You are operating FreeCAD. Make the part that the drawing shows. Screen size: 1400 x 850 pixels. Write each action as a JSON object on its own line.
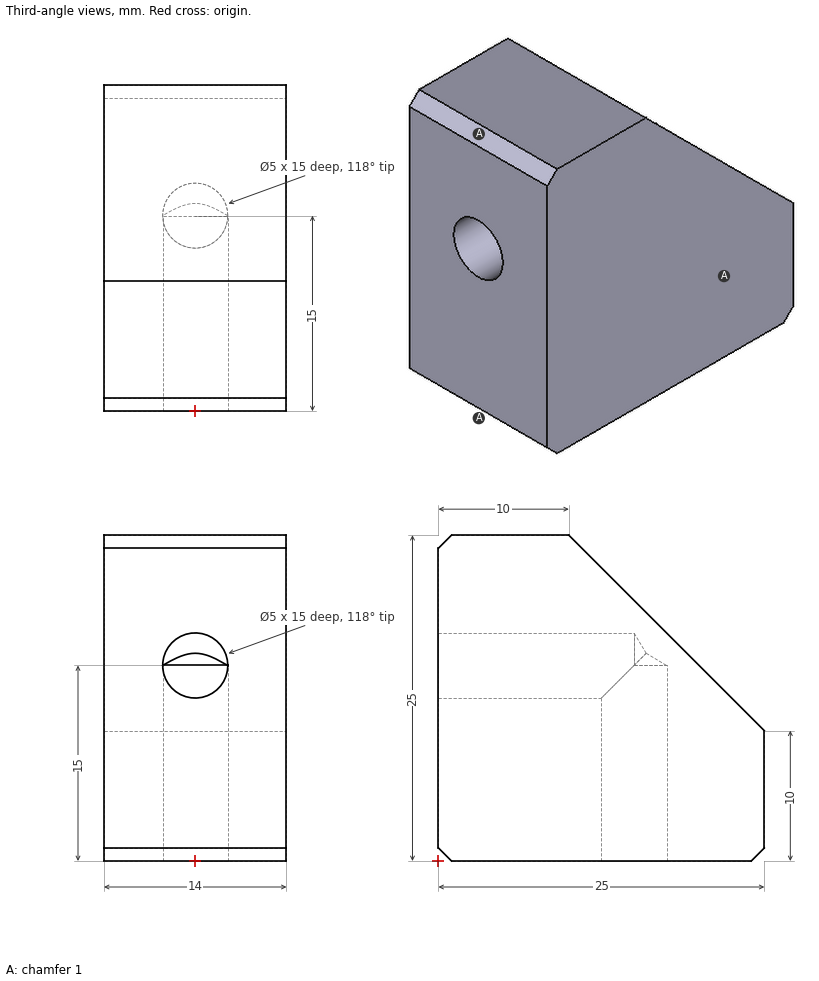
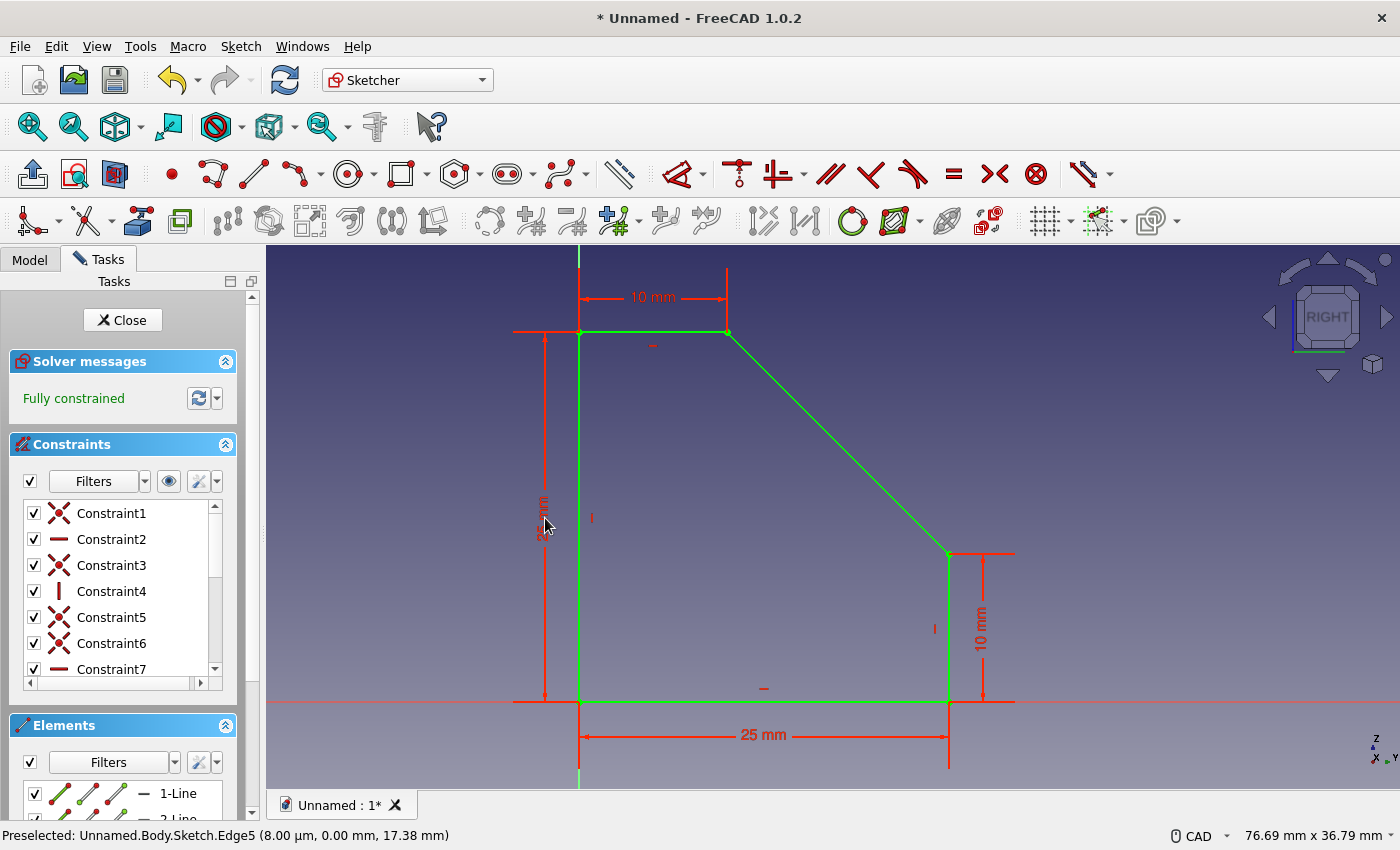
{"action": "left_click", "coordinate": [123, 320]}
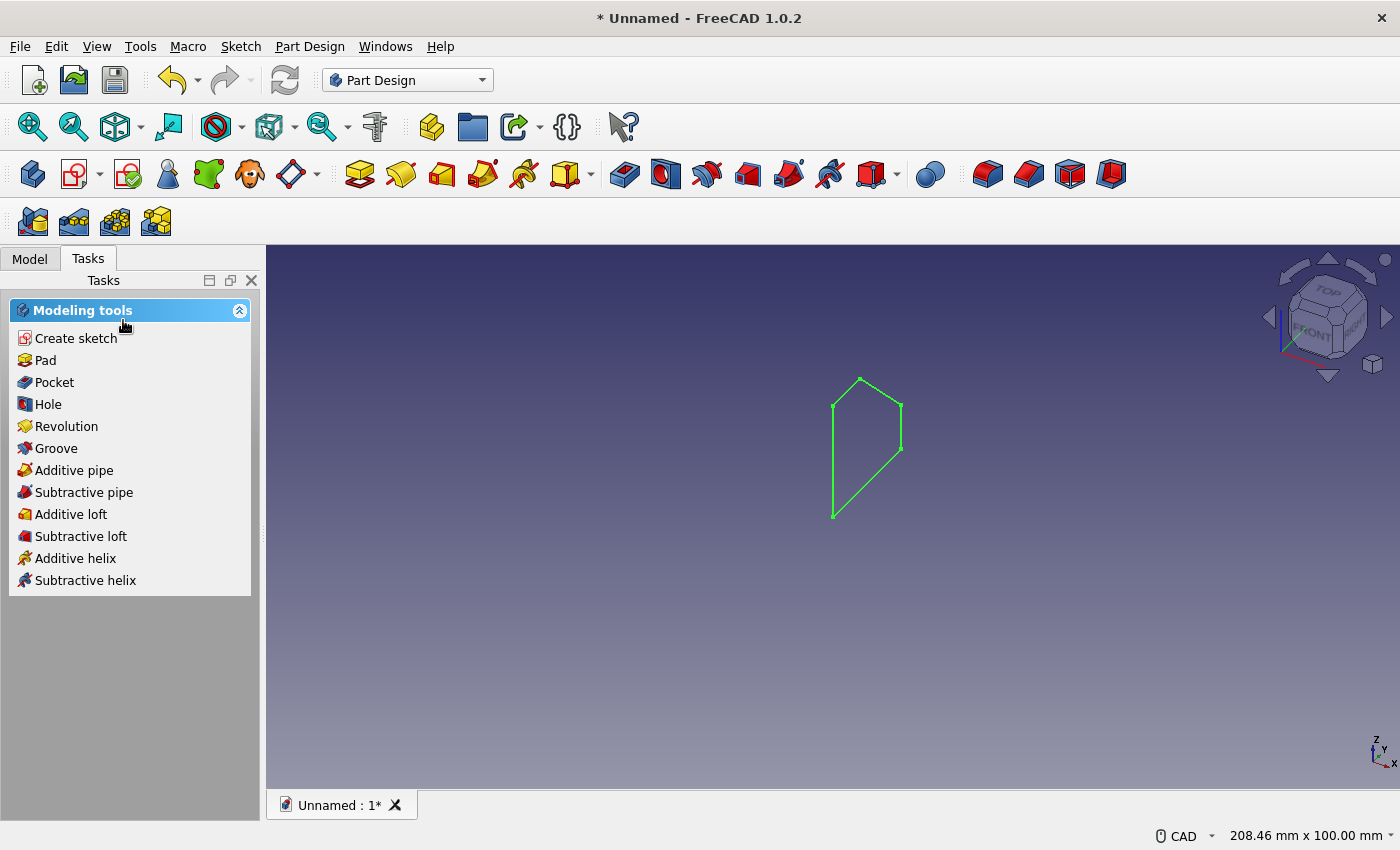
{"action": "left_click", "coordinate": [360, 174]}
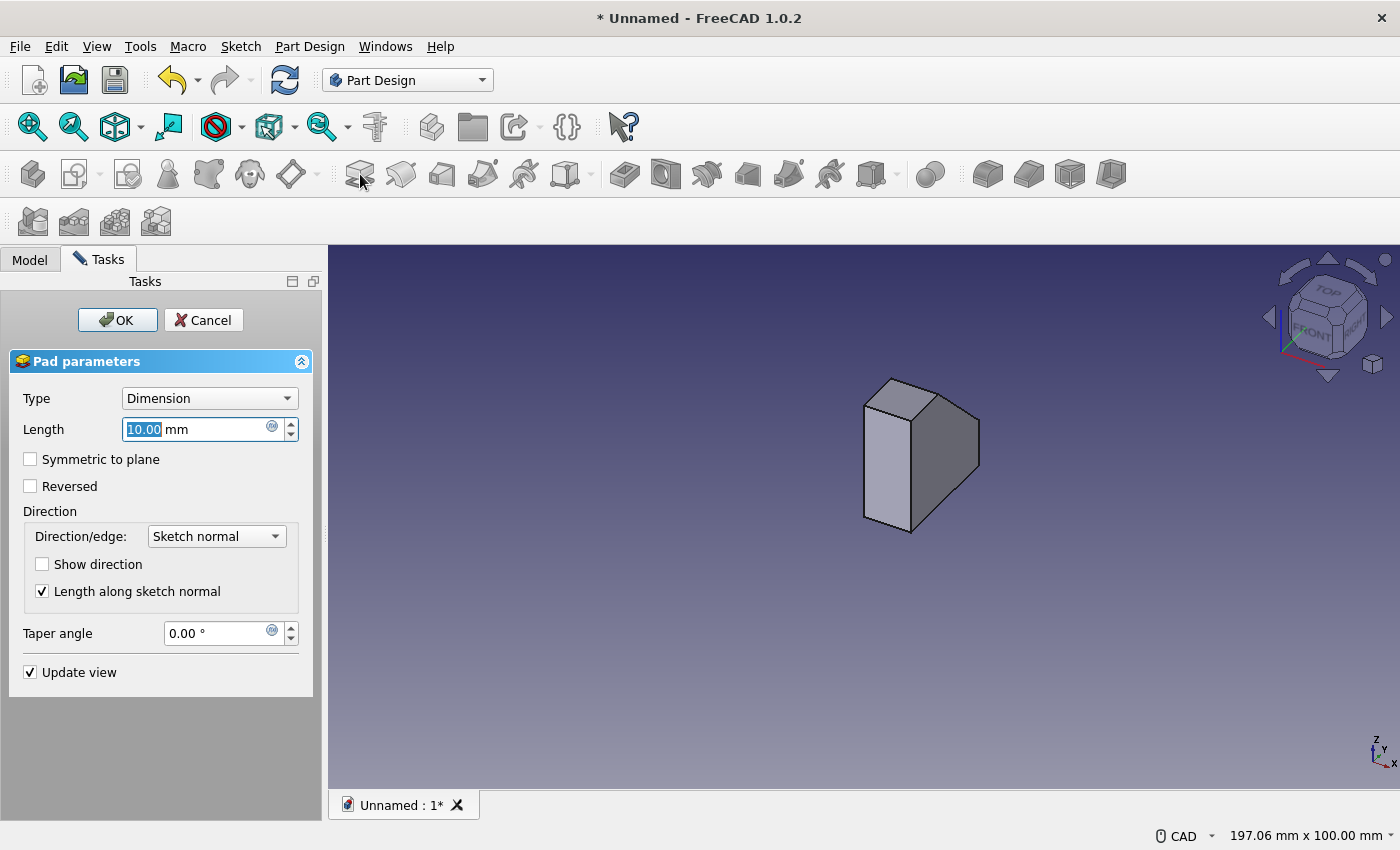
{"action": "type", "text": "14"}
{"action": "key", "text": "Tab"}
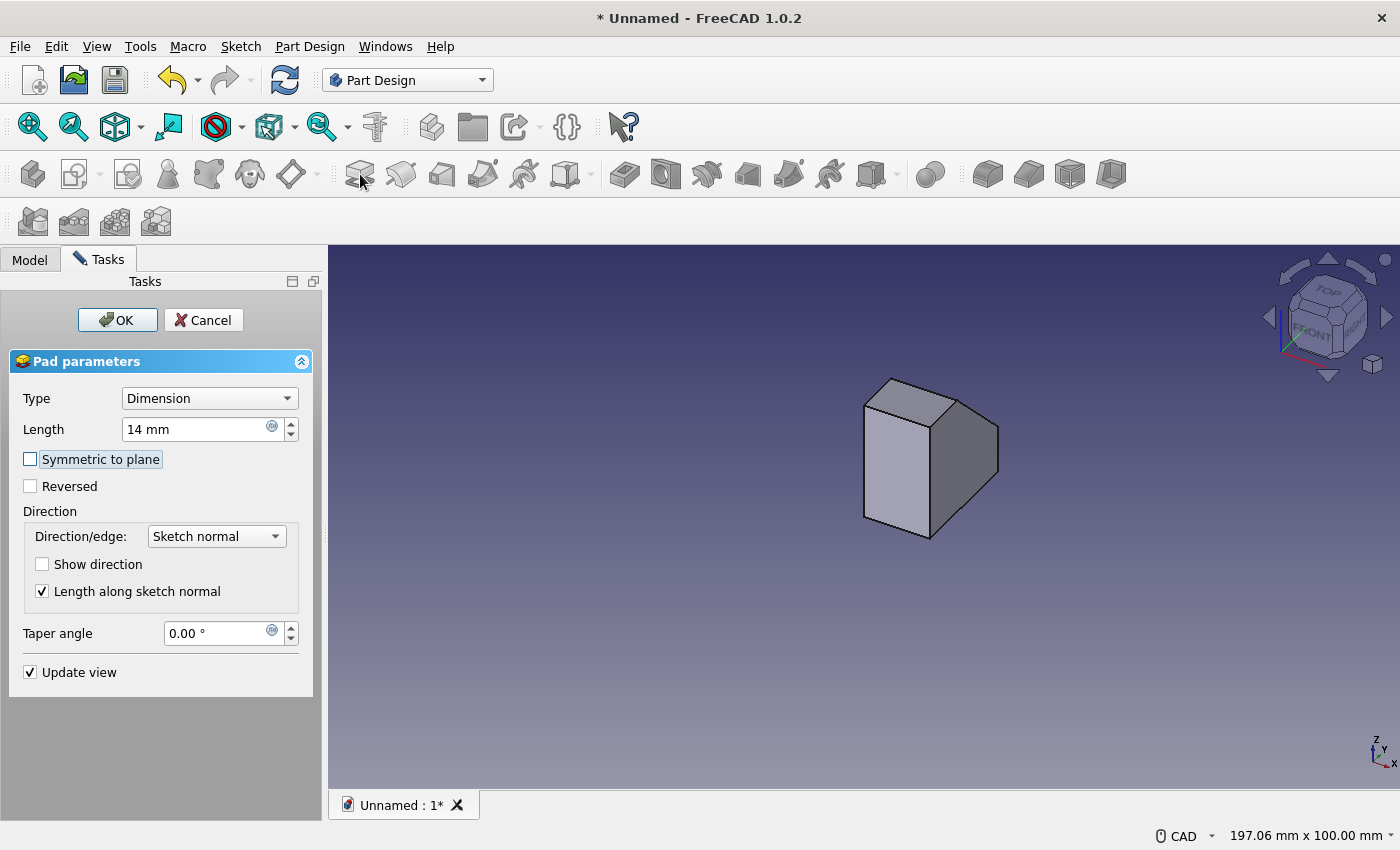
{"action": "left_click", "coordinate": [31, 459]}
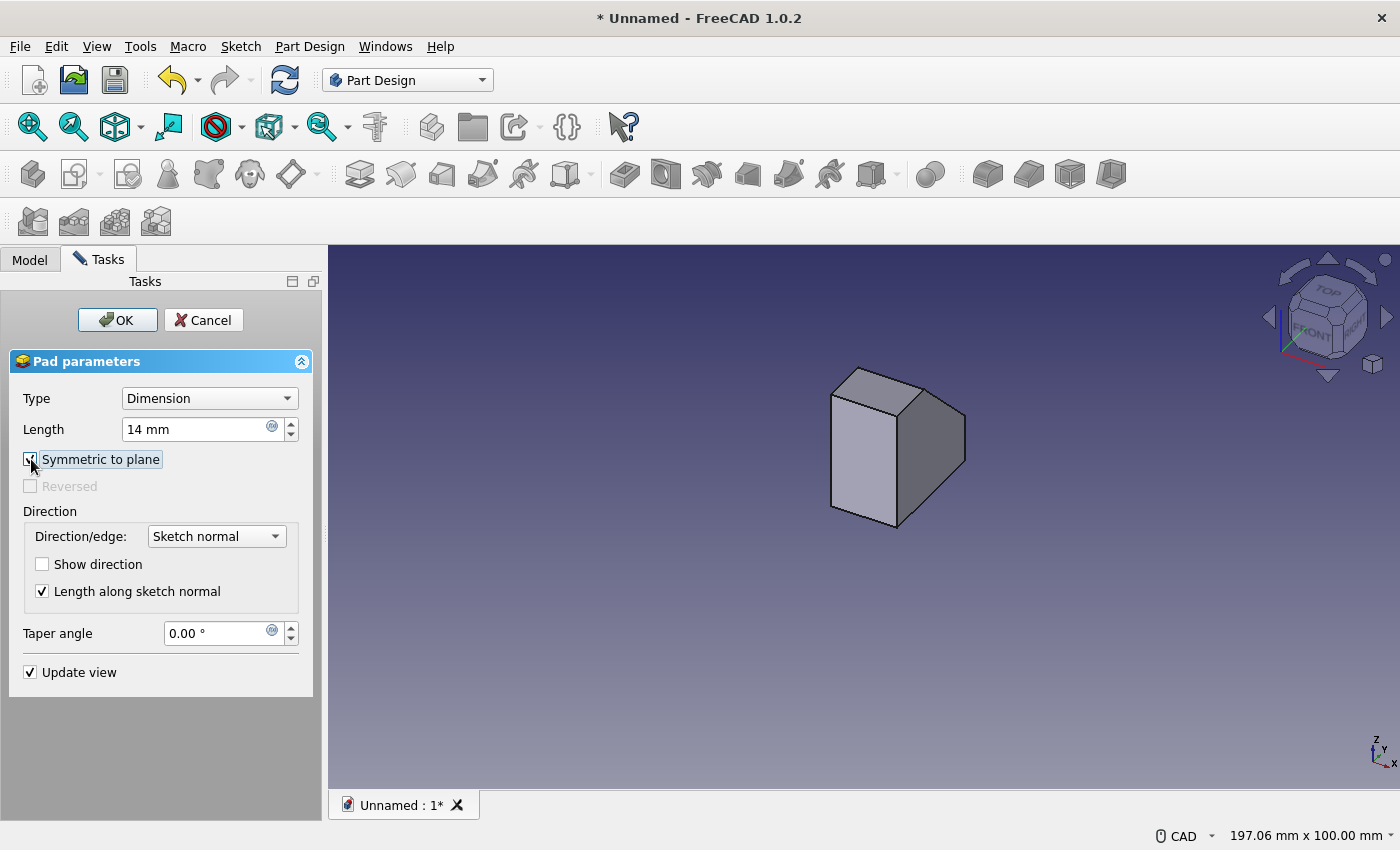
{"action": "left_click", "coordinate": [118, 320]}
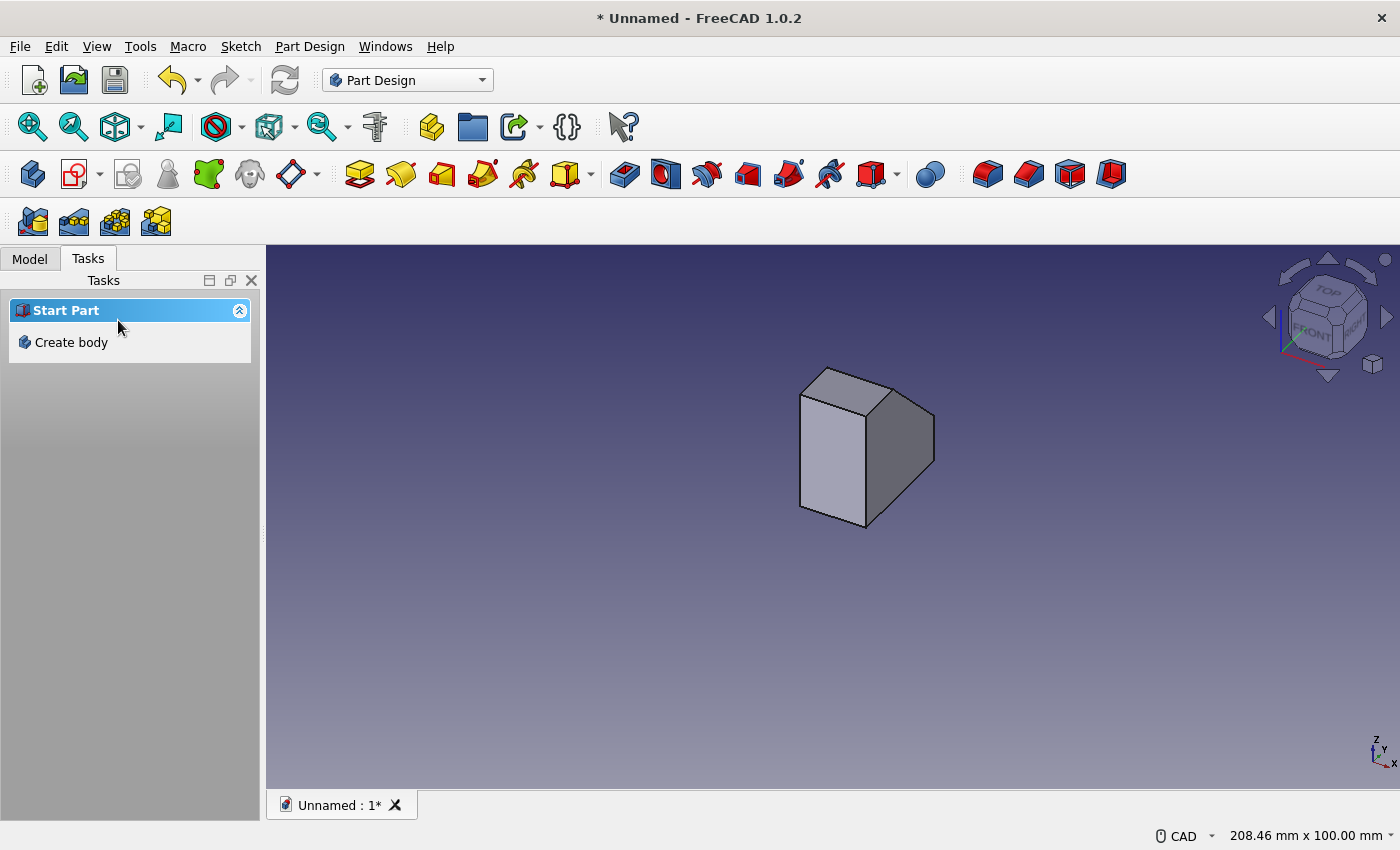
{"action": "left_click", "coordinate": [33, 128]}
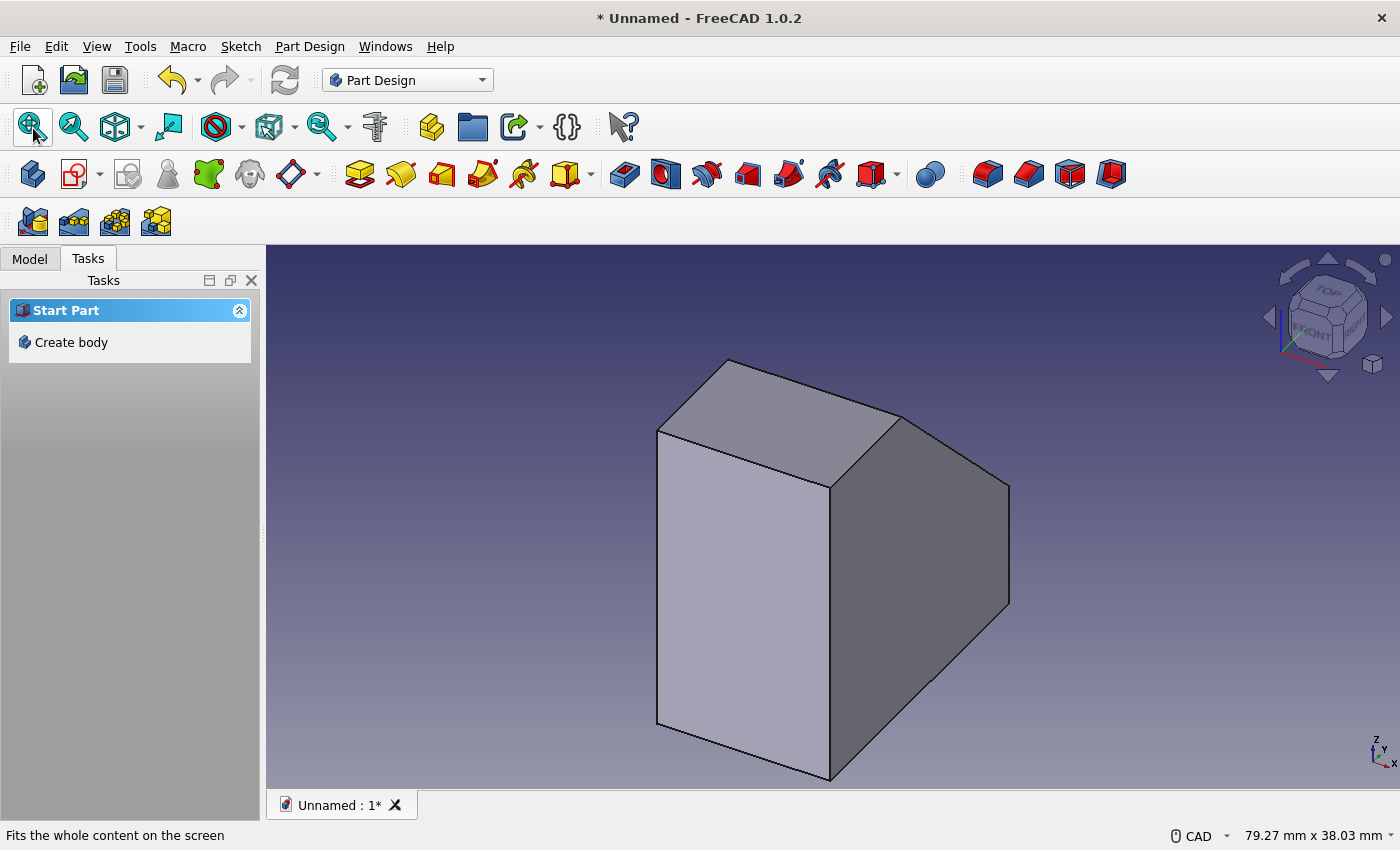
{"action": "left_click", "coordinate": [744, 647]}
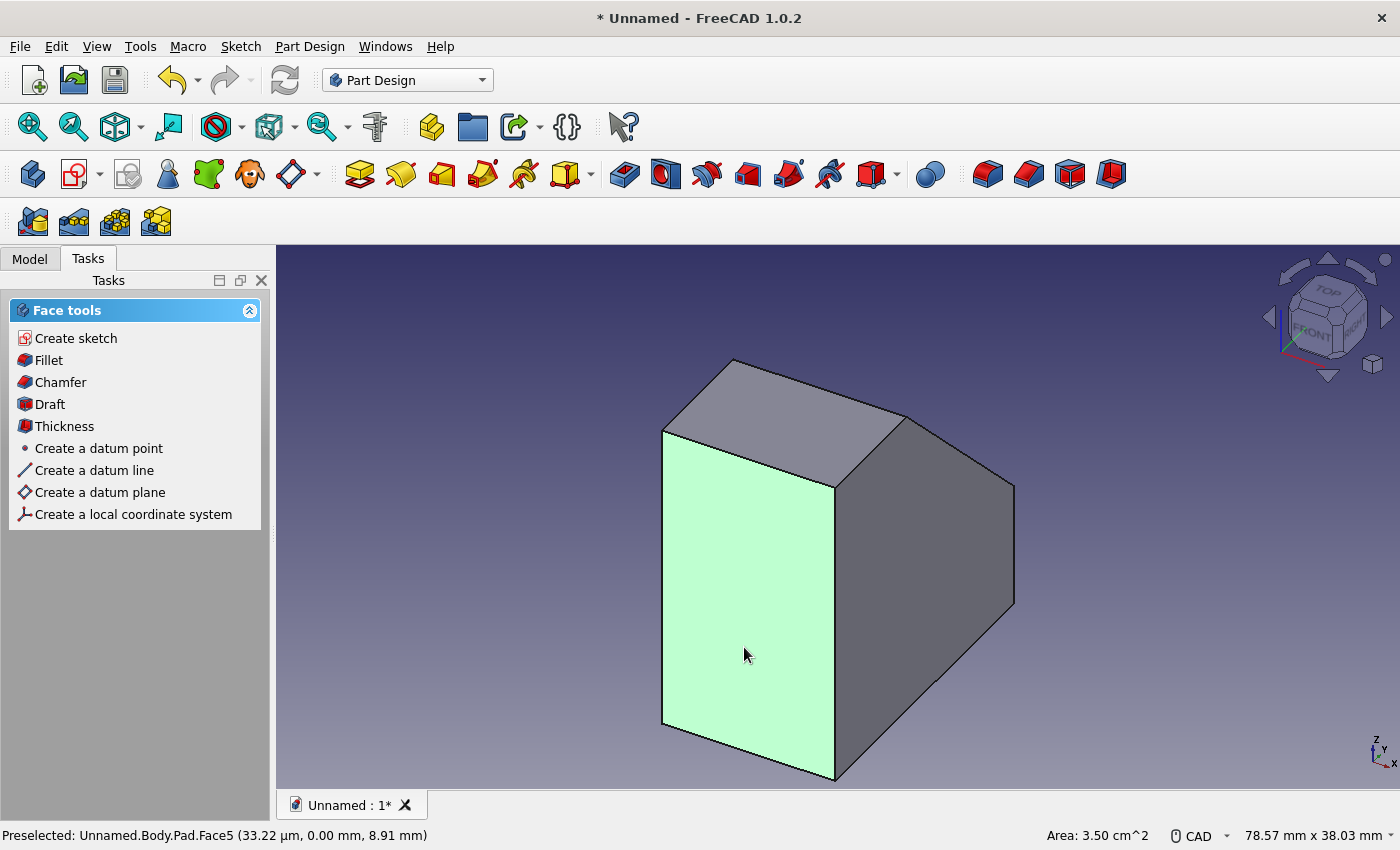
{"action": "left_click", "coordinate": [74, 174]}